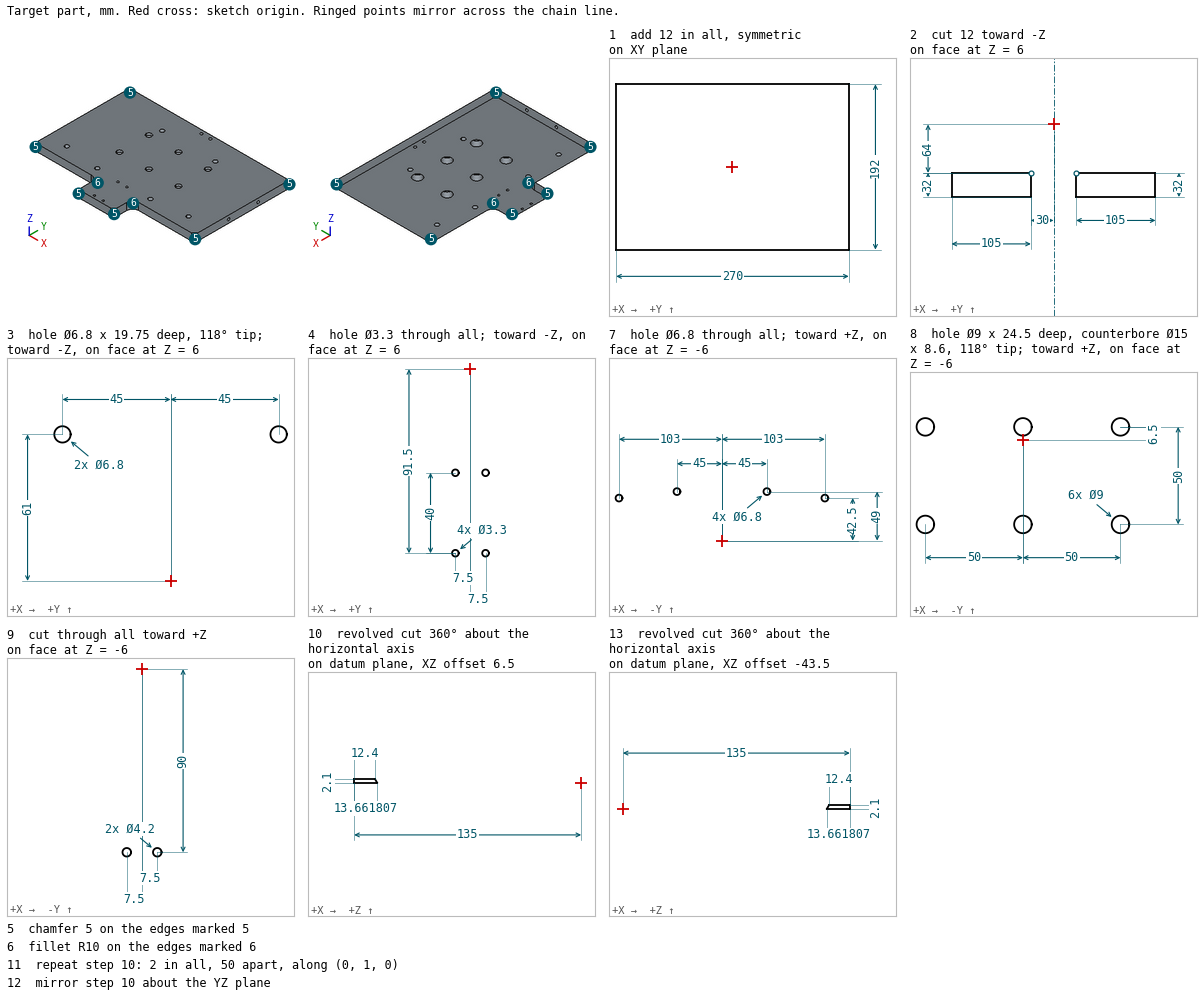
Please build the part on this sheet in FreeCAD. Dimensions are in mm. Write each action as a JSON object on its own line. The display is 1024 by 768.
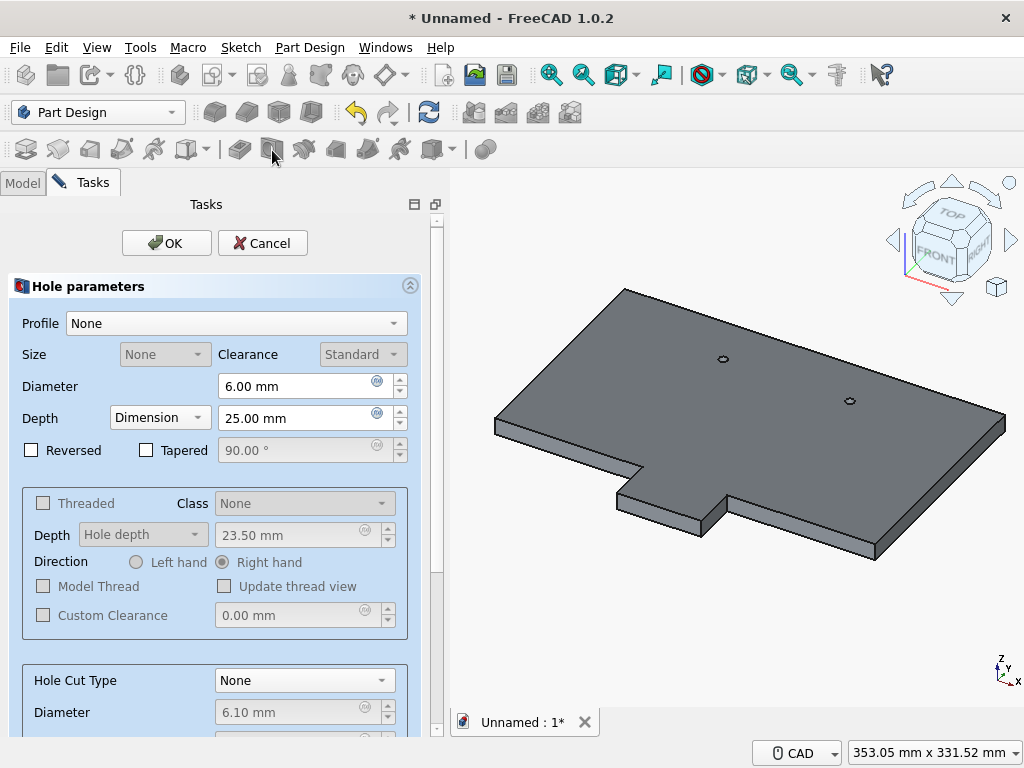
{"action": "triple_click", "coordinate": [305, 386]}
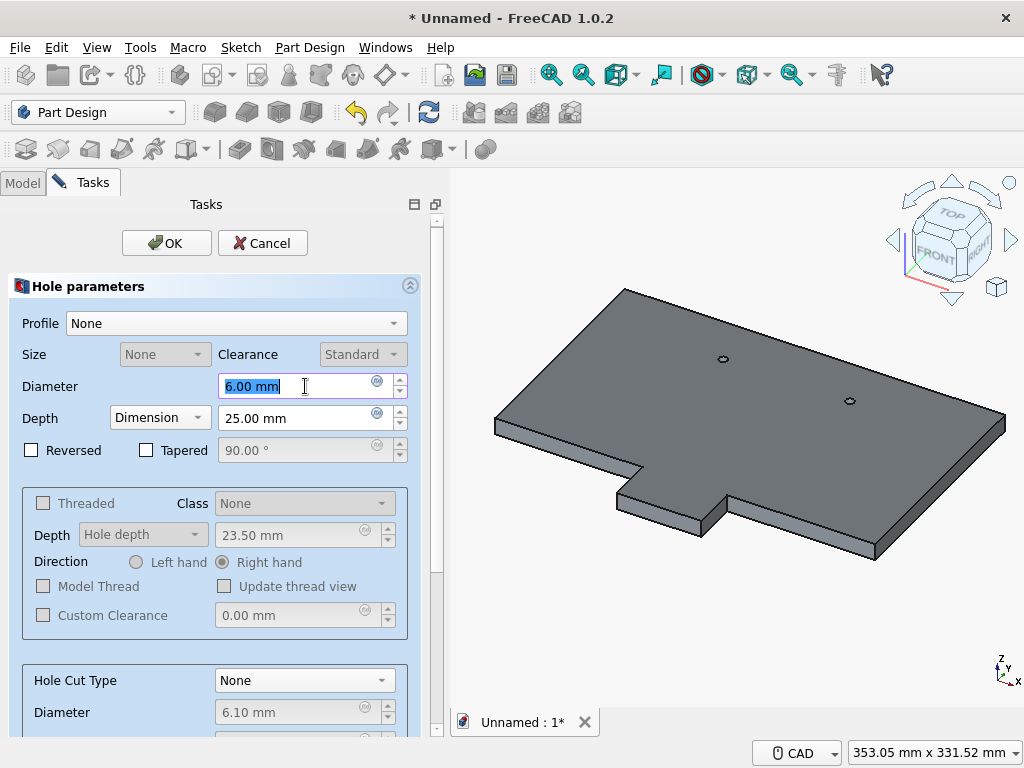
{"action": "type", "text": "6.8"}
{"action": "key", "text": "Tab"}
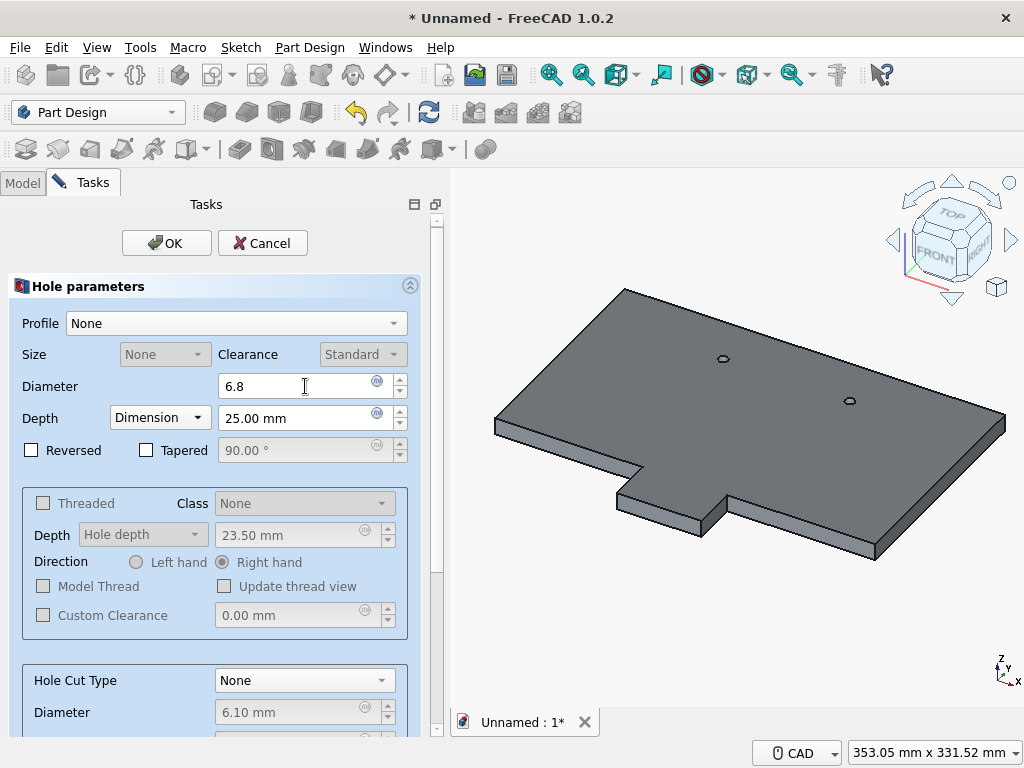
{"action": "triple_click", "coordinate": [305, 418]}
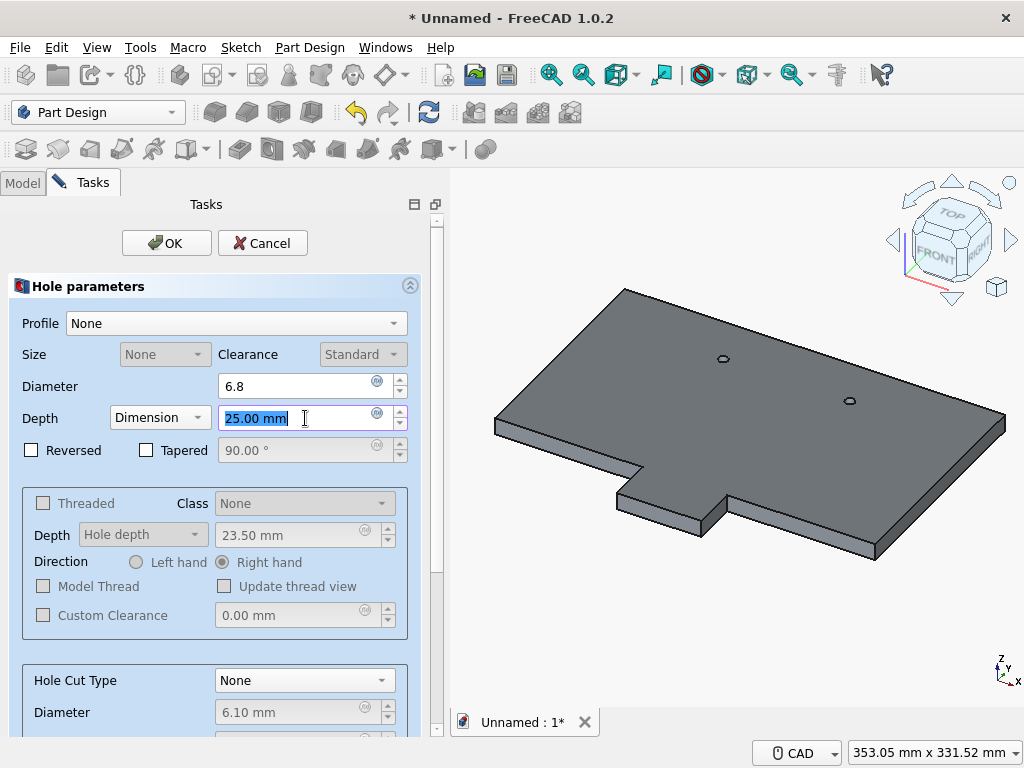
{"action": "type", "text": "19.75"}
{"action": "key", "text": "Tab"}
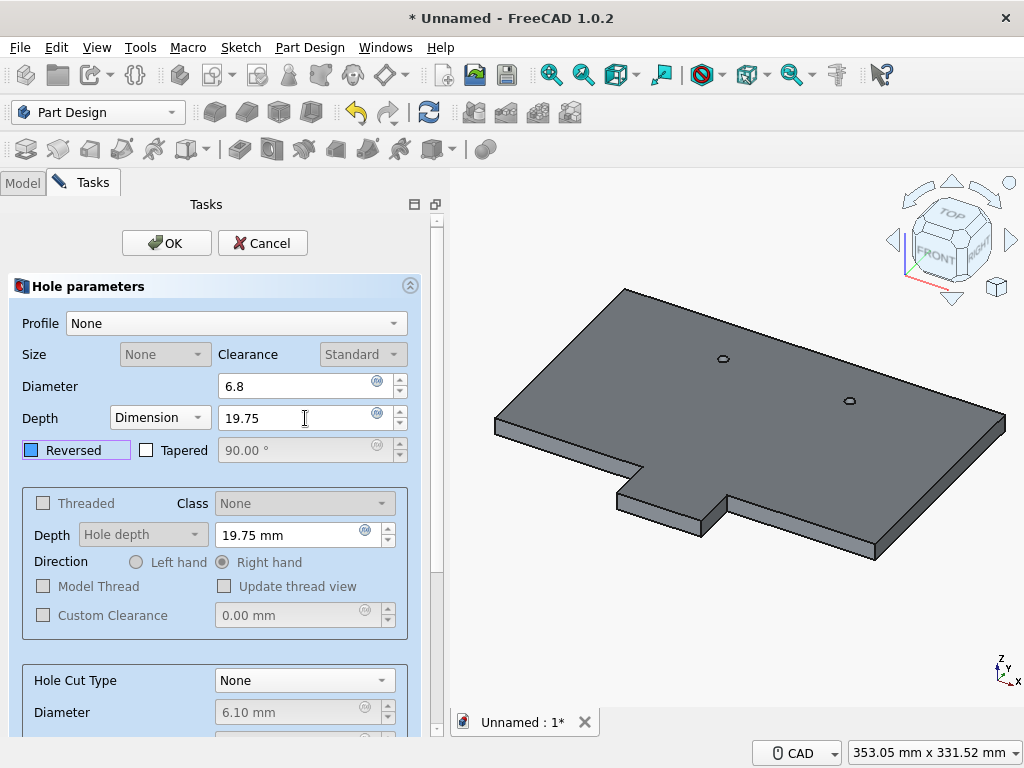
{"action": "left_click", "coordinate": [167, 243]}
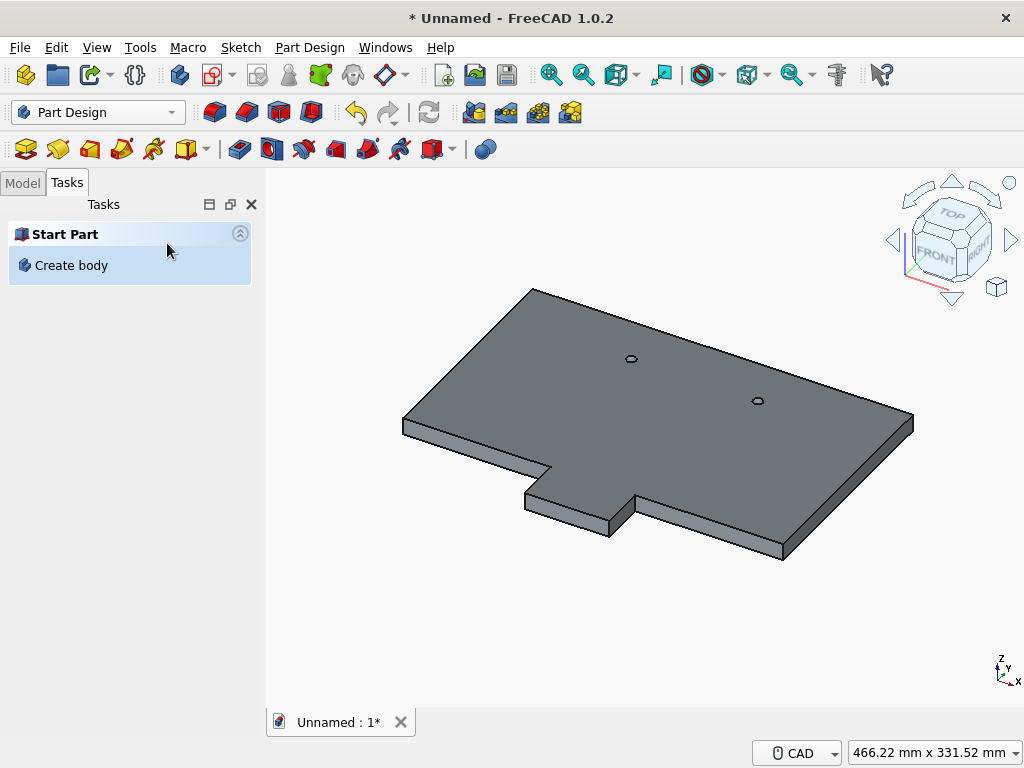
{"action": "left_click", "coordinate": [645, 429]}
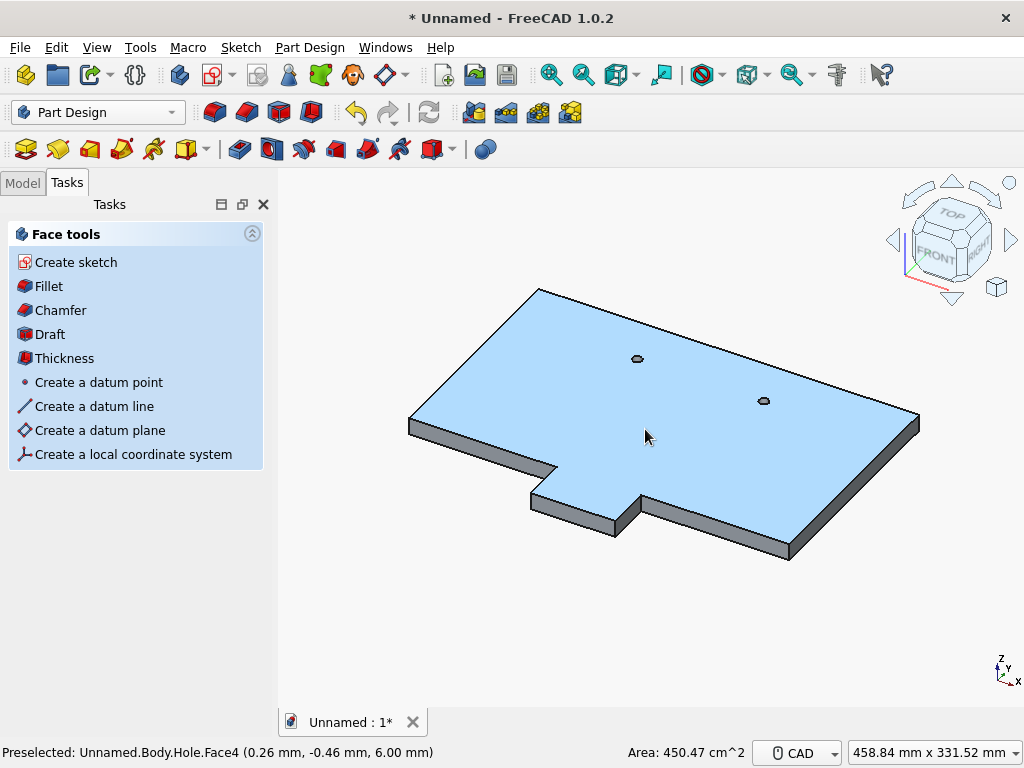
{"action": "left_click", "coordinate": [212, 76]}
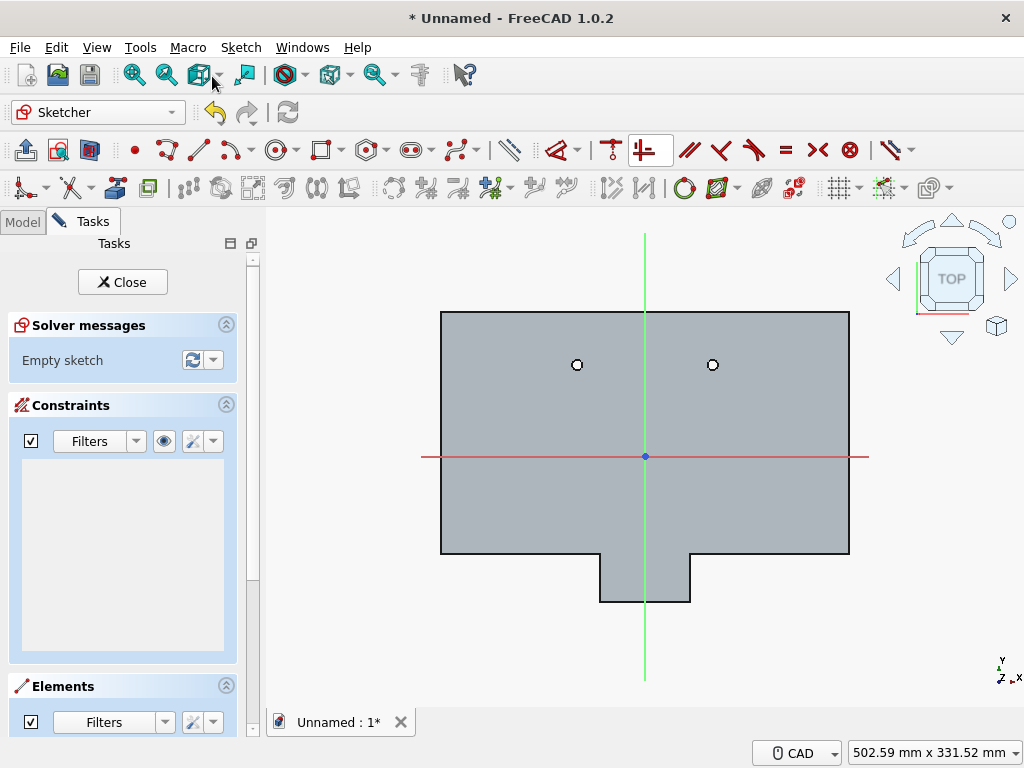
{"action": "scroll", "coordinate": [701, 585], "scroll_direction": "up", "scroll_amount": 4}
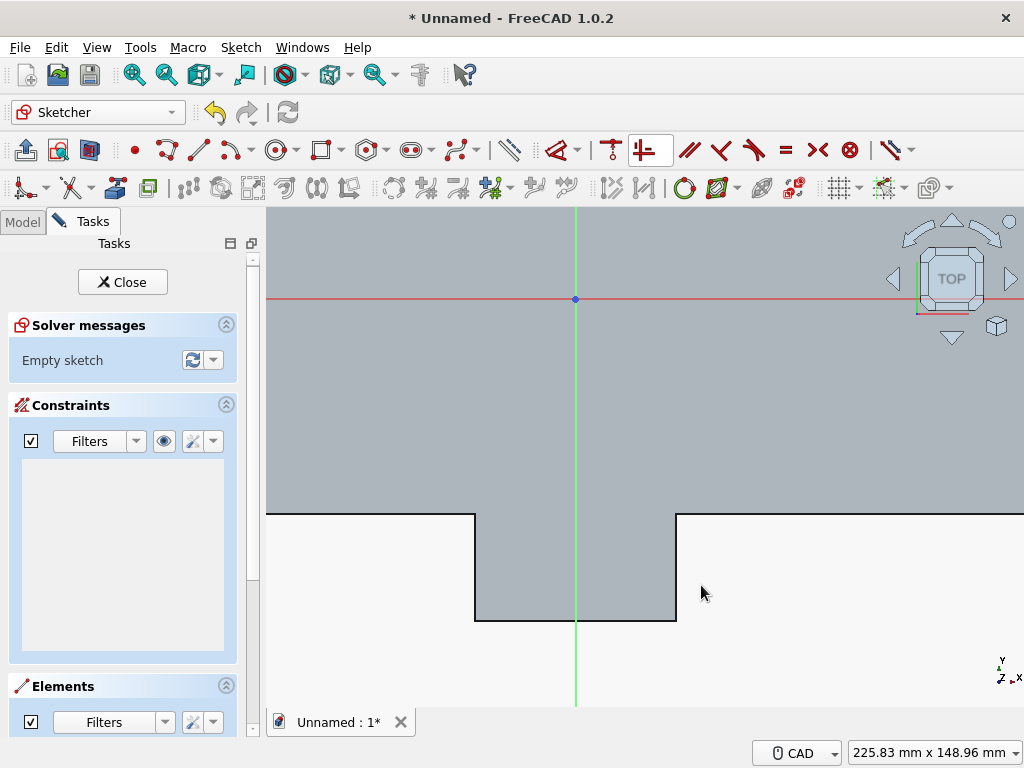
{"action": "key", "text": "g c"}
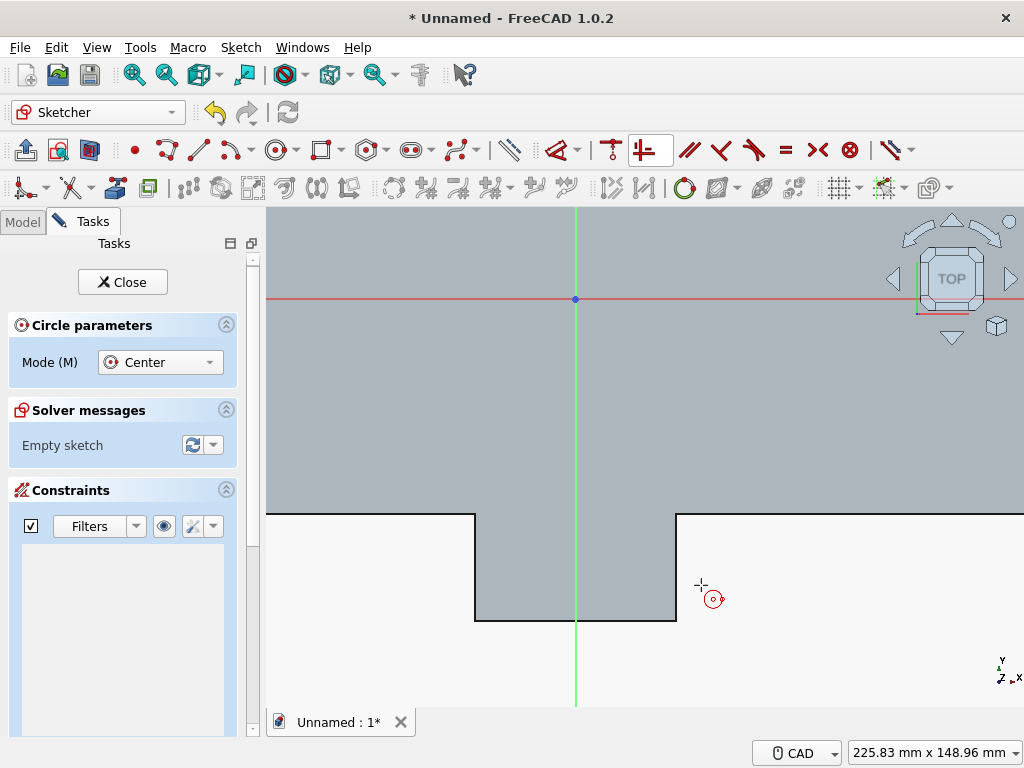
{"action": "scroll", "coordinate": [550, 606], "scroll_direction": "up", "scroll_amount": 8}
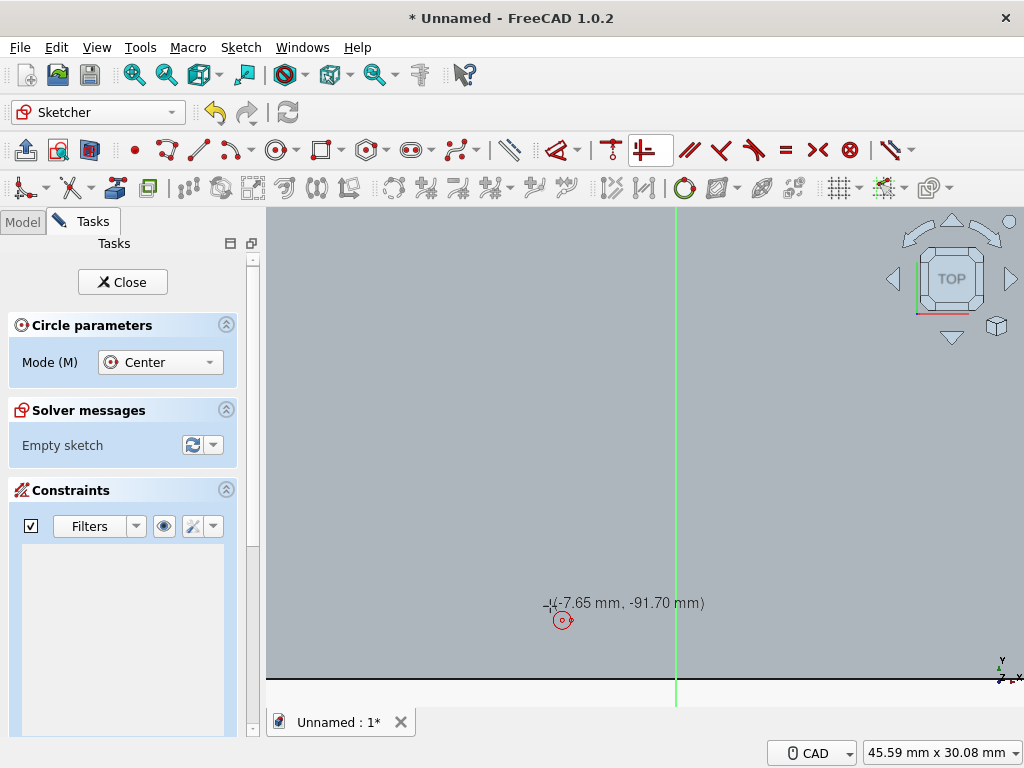
{"action": "scroll", "coordinate": [551, 609], "scroll_direction": "down", "scroll_amount": 8}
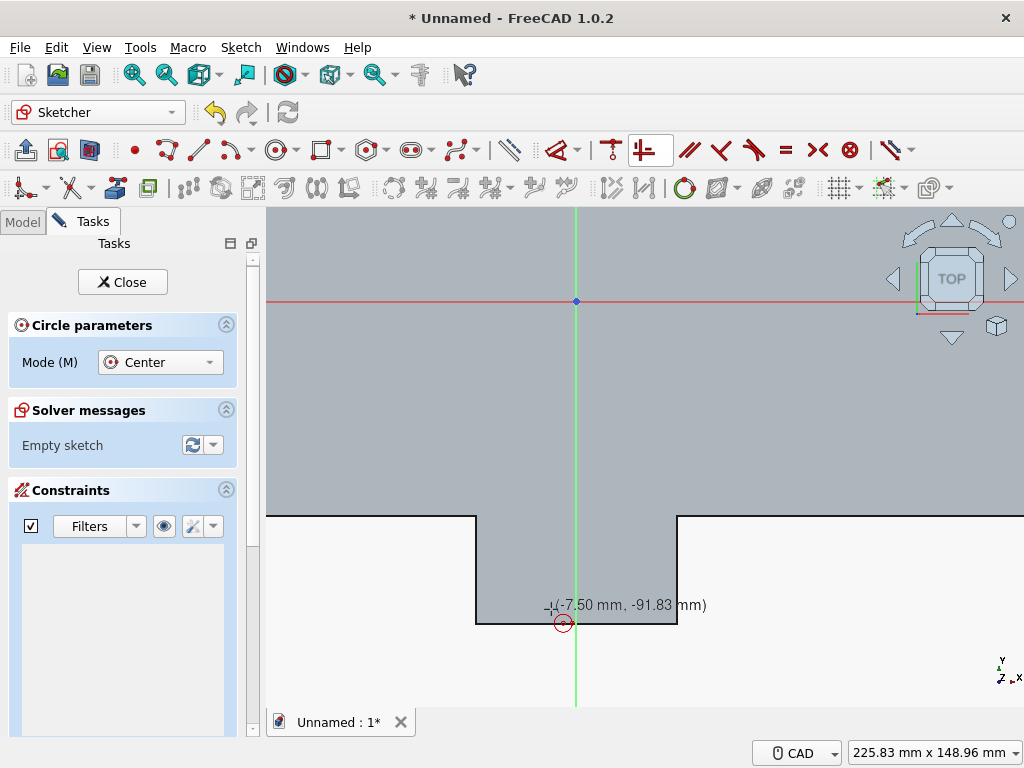
{"action": "left_click", "coordinate": [551, 609]}
{"action": "mouse_move", "coordinate": [555, 605]}